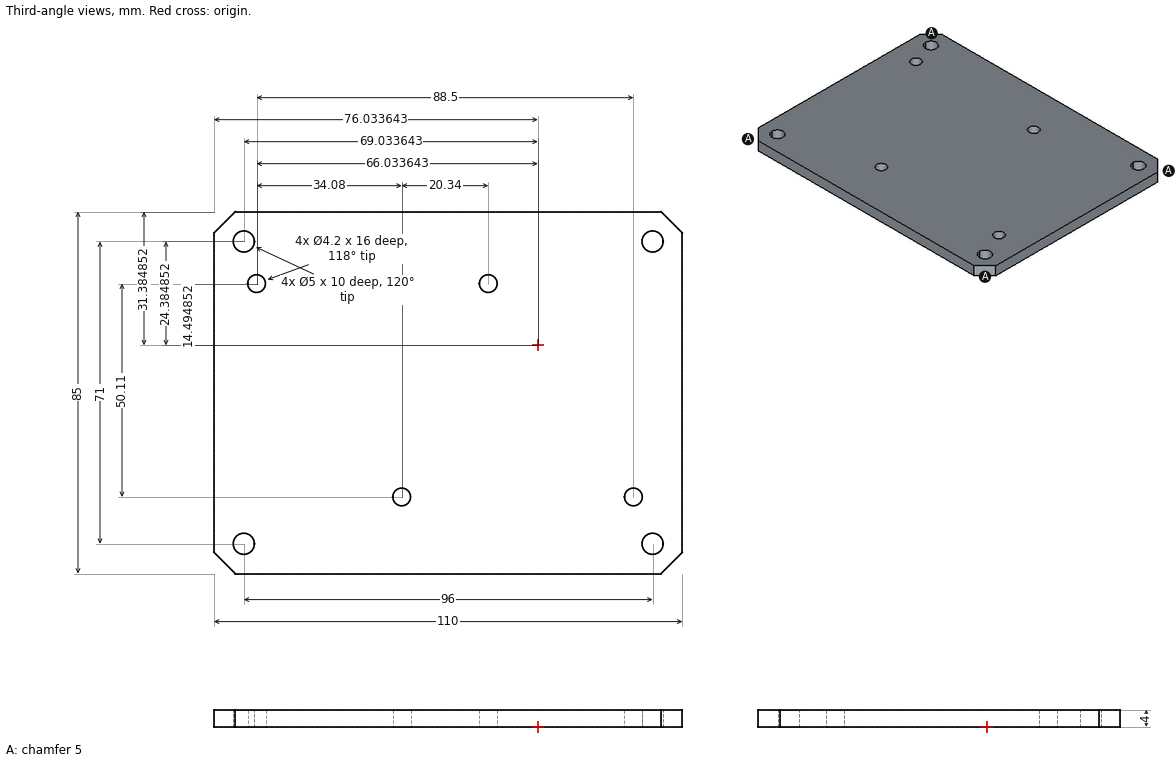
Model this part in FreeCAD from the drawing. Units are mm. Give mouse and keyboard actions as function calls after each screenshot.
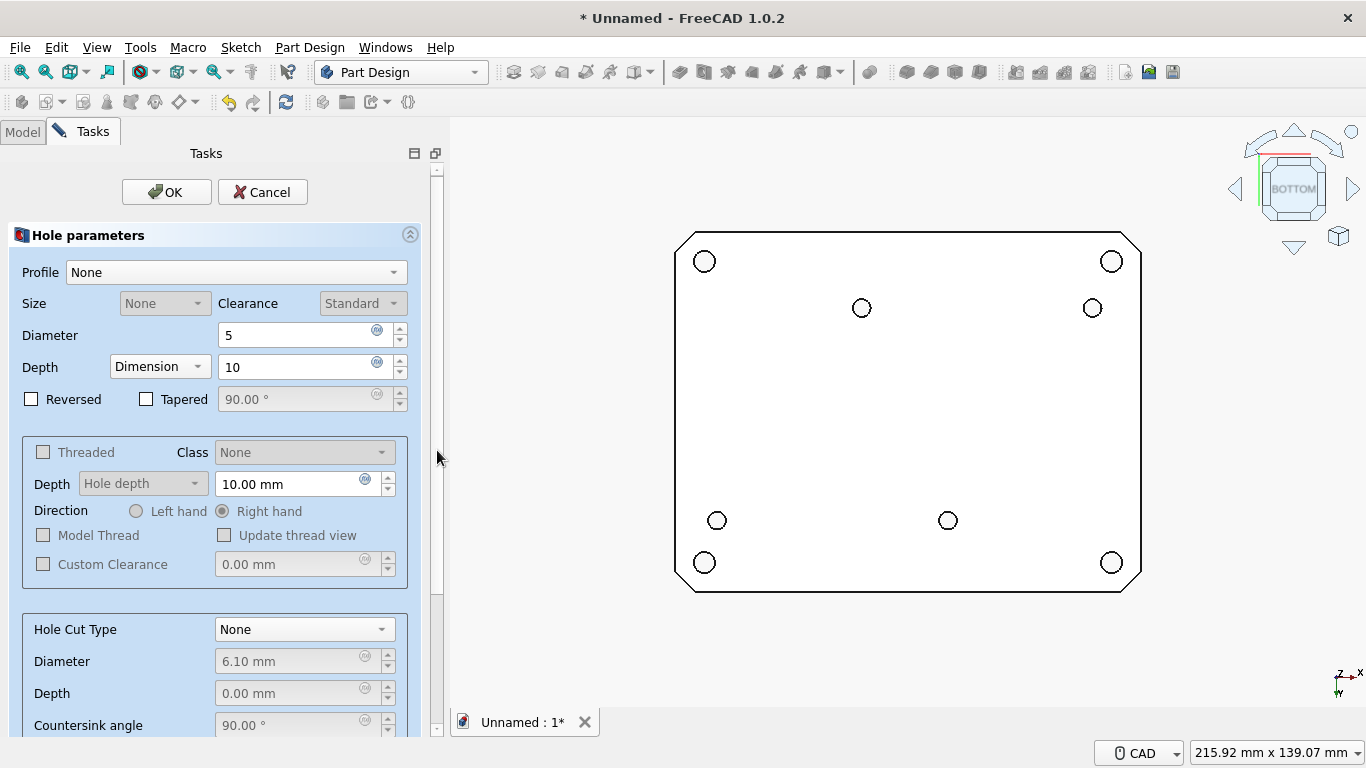
click(167, 192)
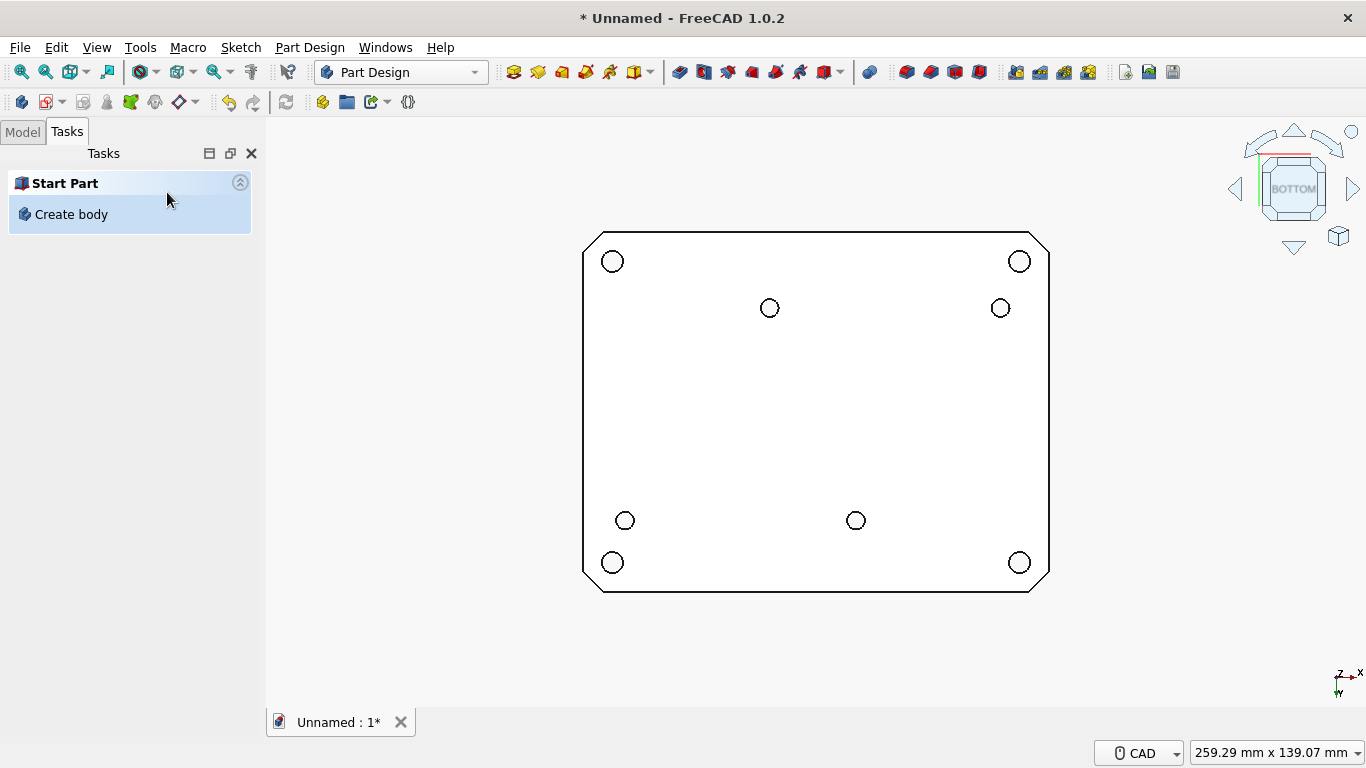
key(0)